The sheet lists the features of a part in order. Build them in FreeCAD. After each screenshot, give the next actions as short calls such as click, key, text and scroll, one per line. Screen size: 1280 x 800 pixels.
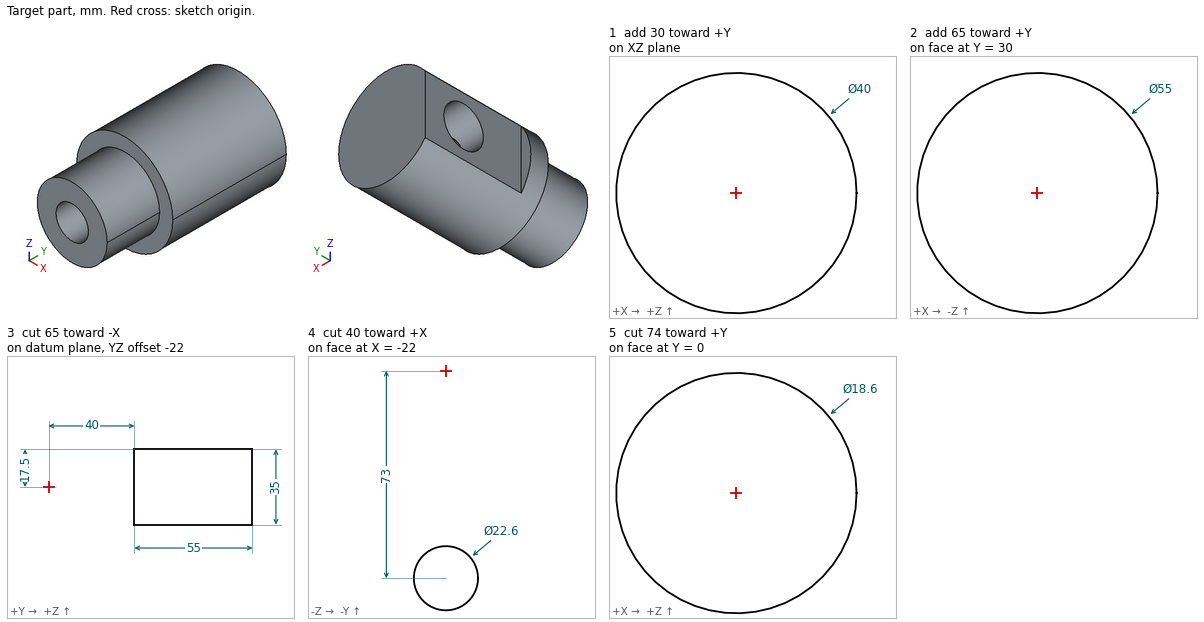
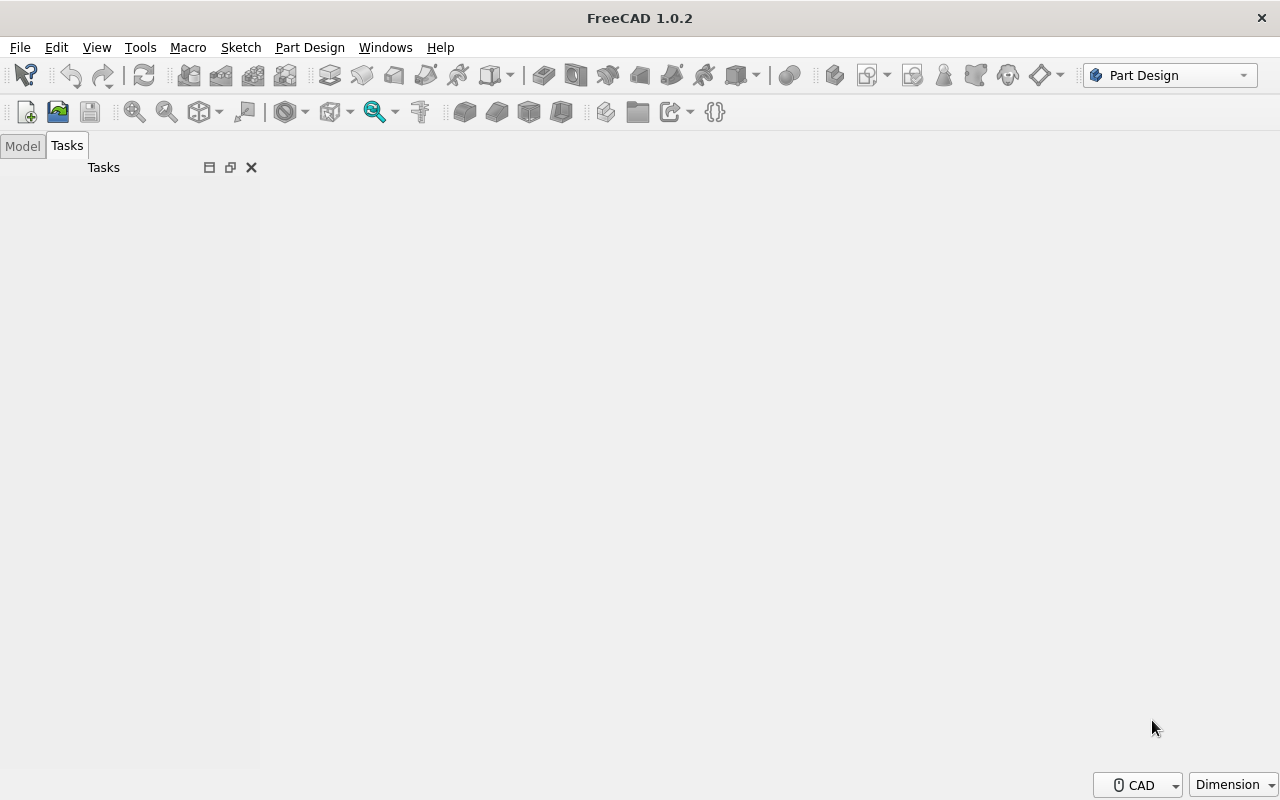
key(ctrl+n)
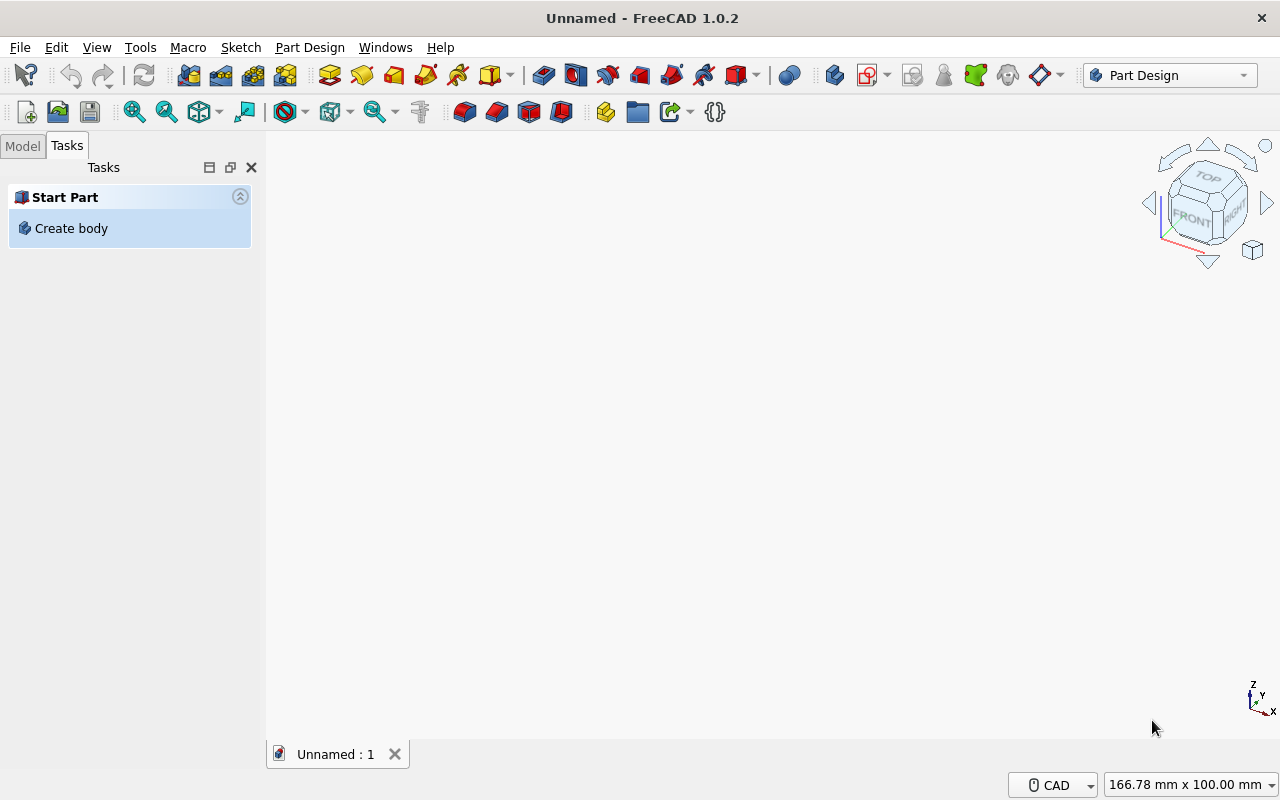
click(868, 76)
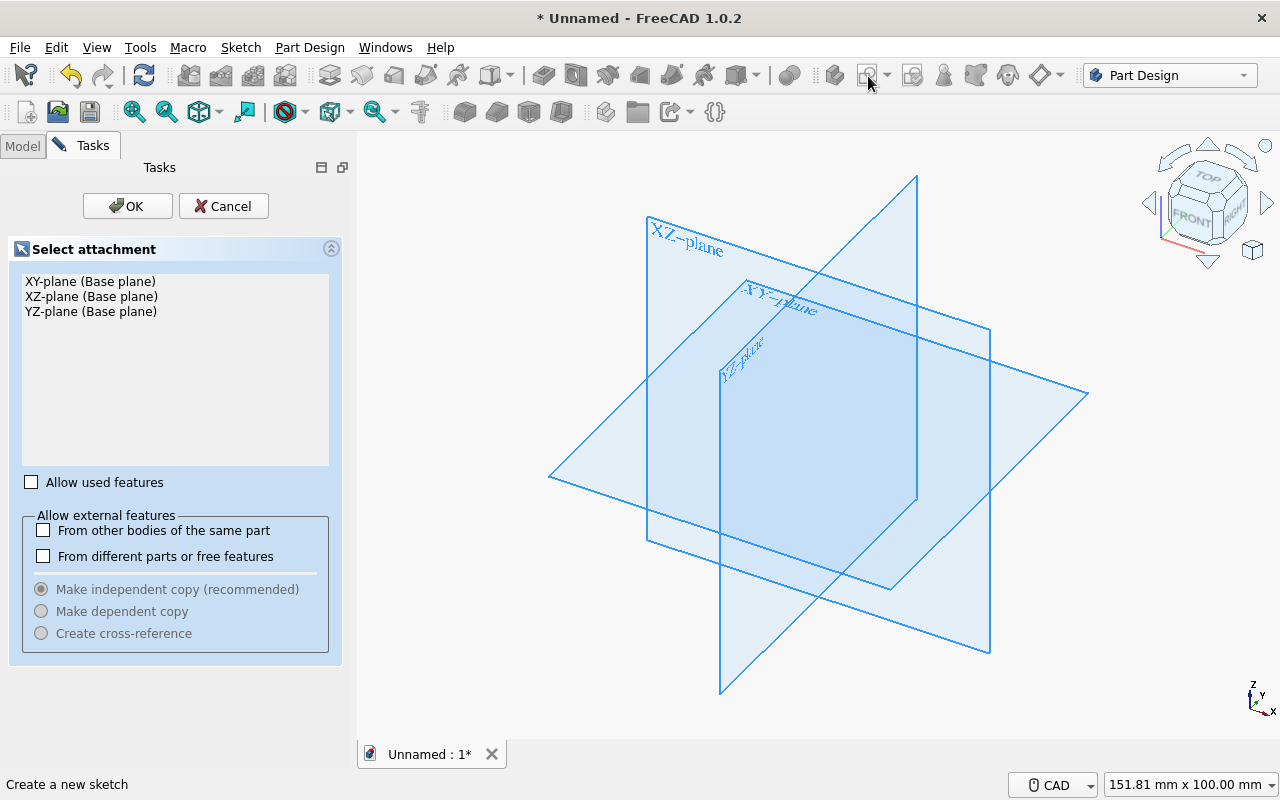
click(82, 296)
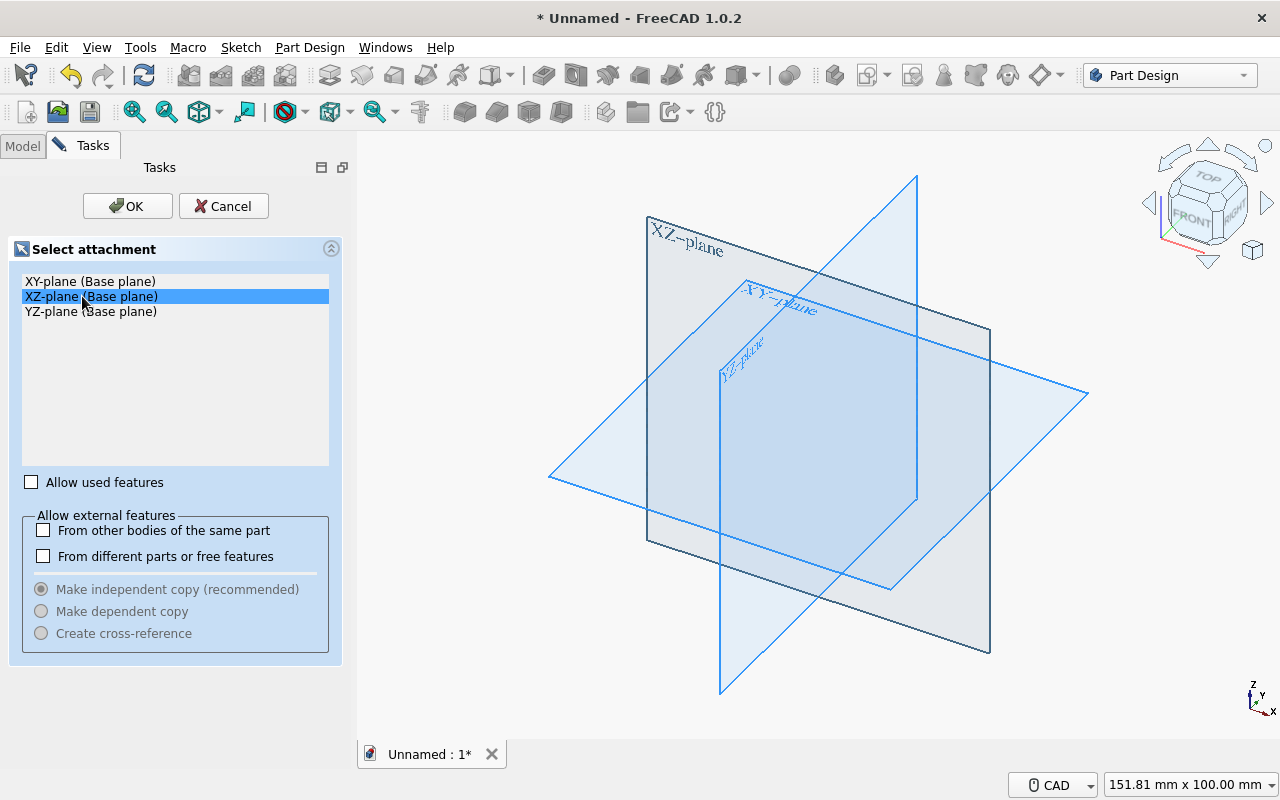
click(128, 206)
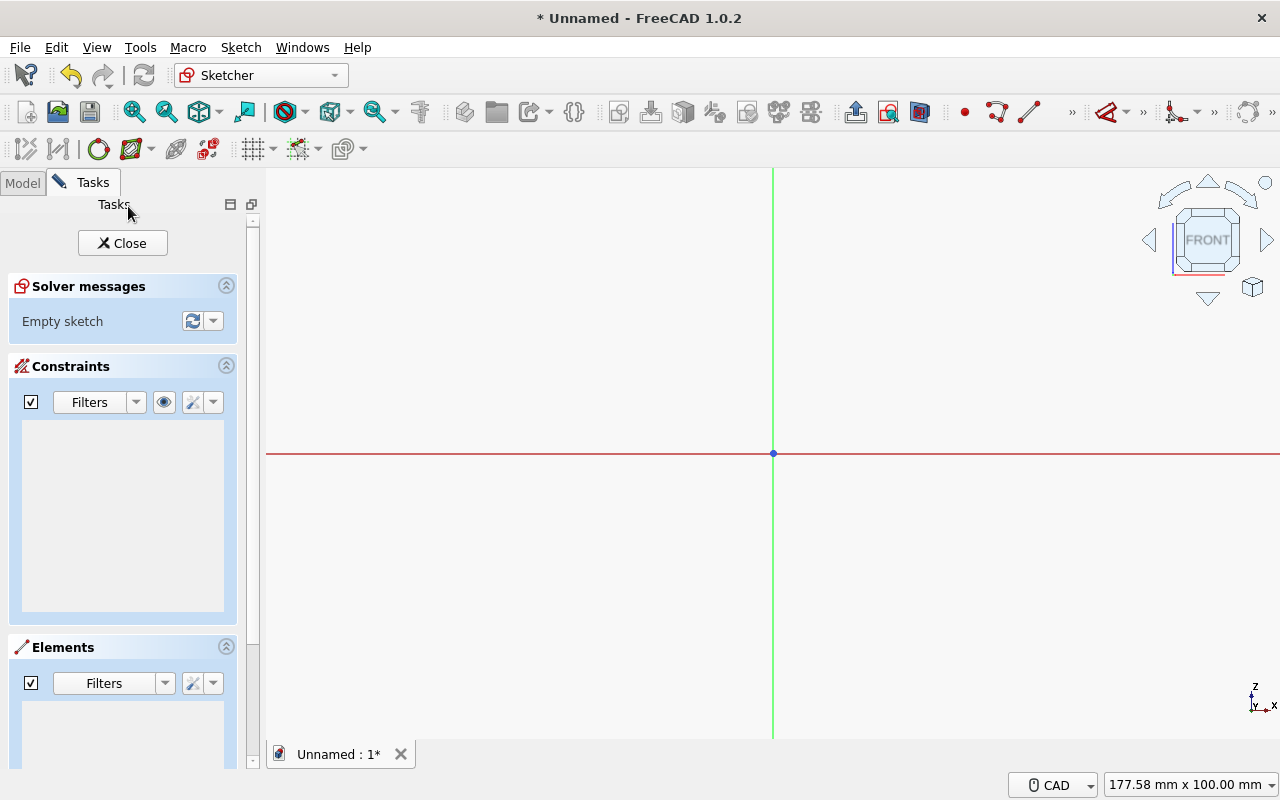
scroll(912, 454, up, 2)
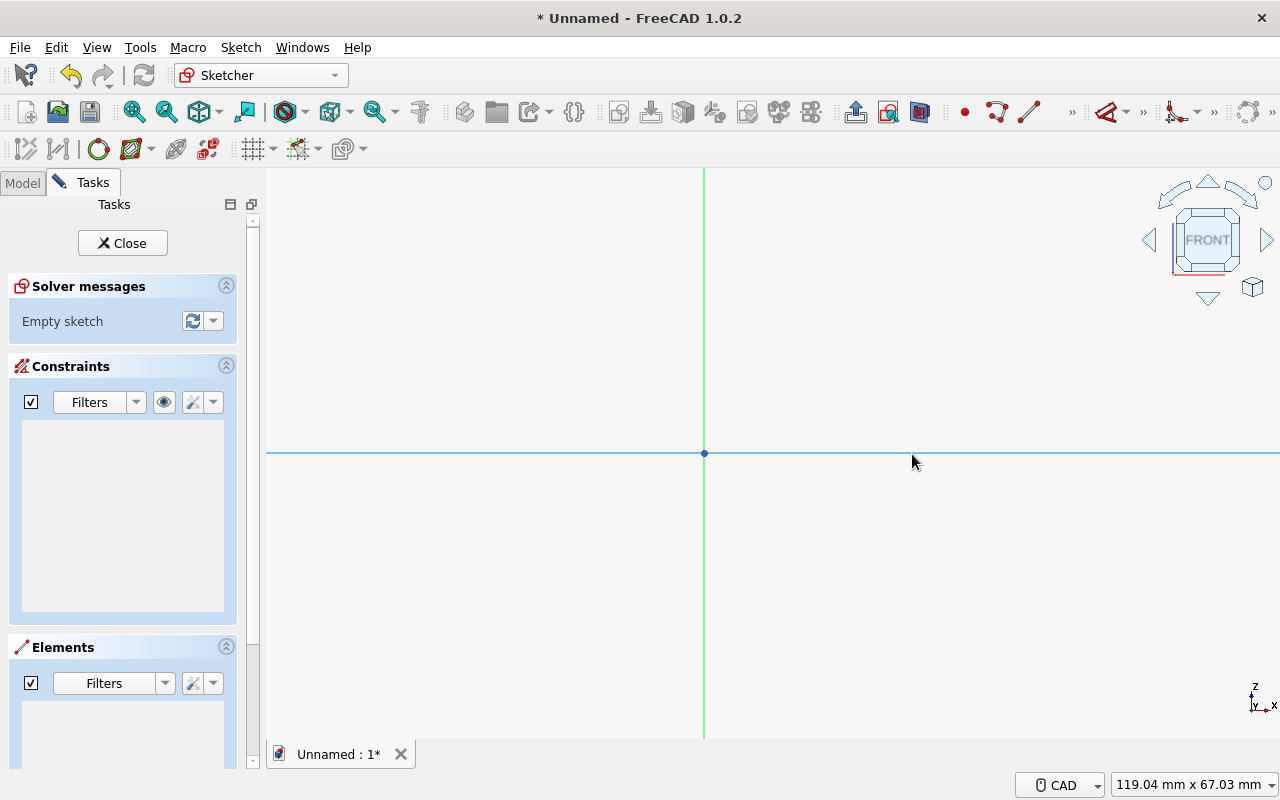
key(g)
key(c)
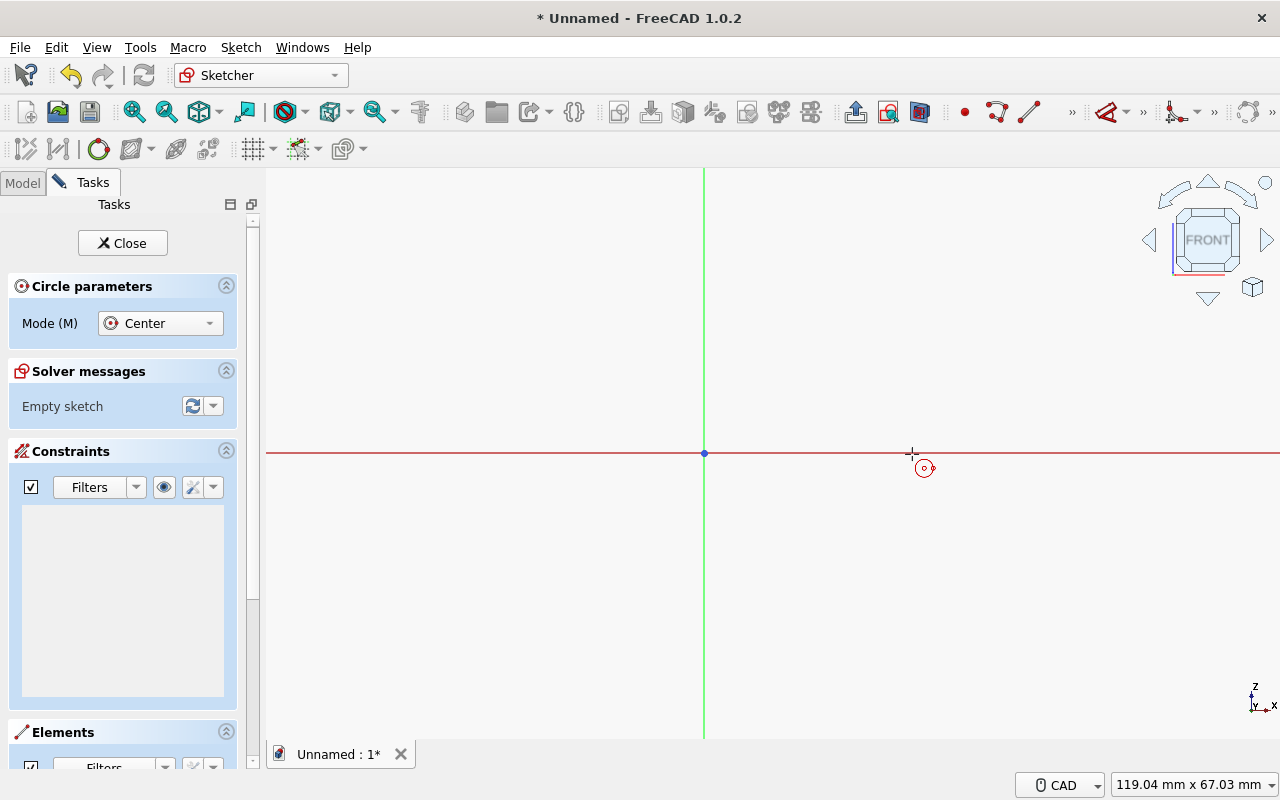
click(704, 453)
move(825, 333)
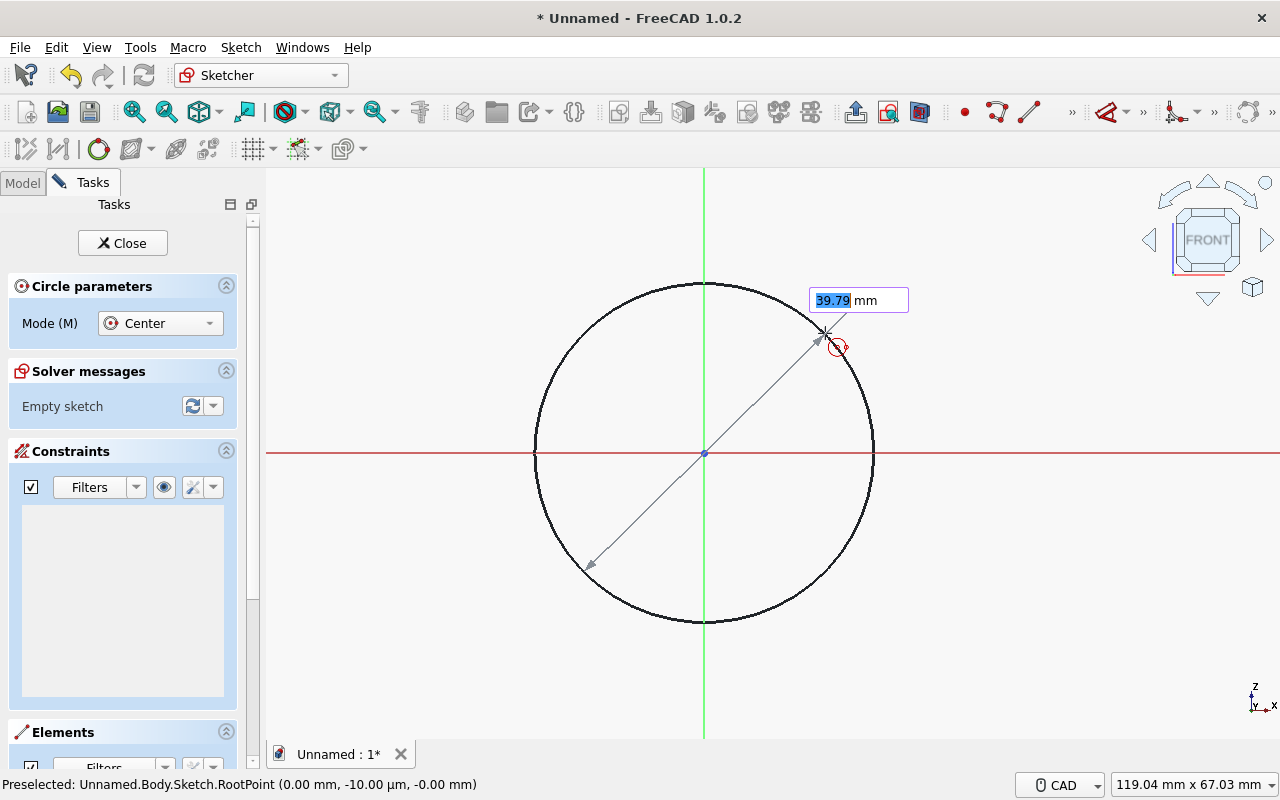
text(40)
key(Return)
key(Escape)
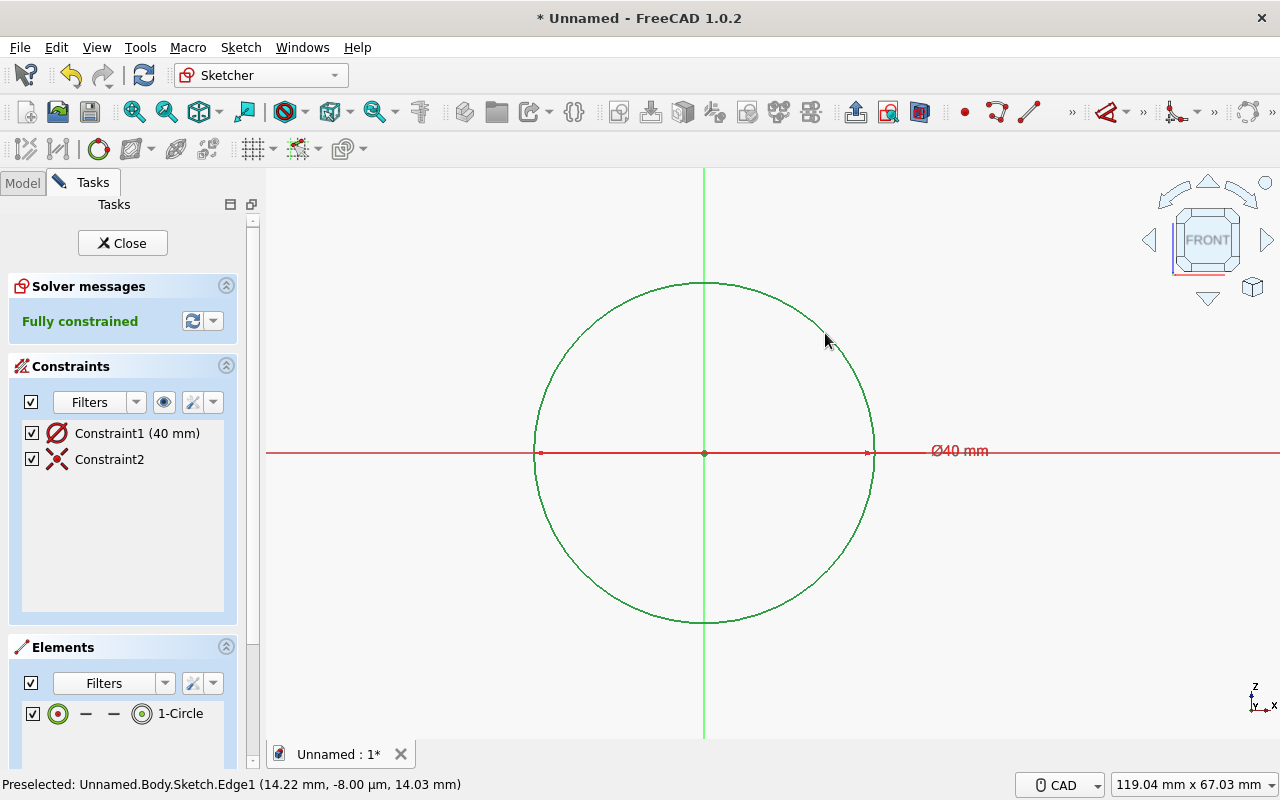
click(123, 243)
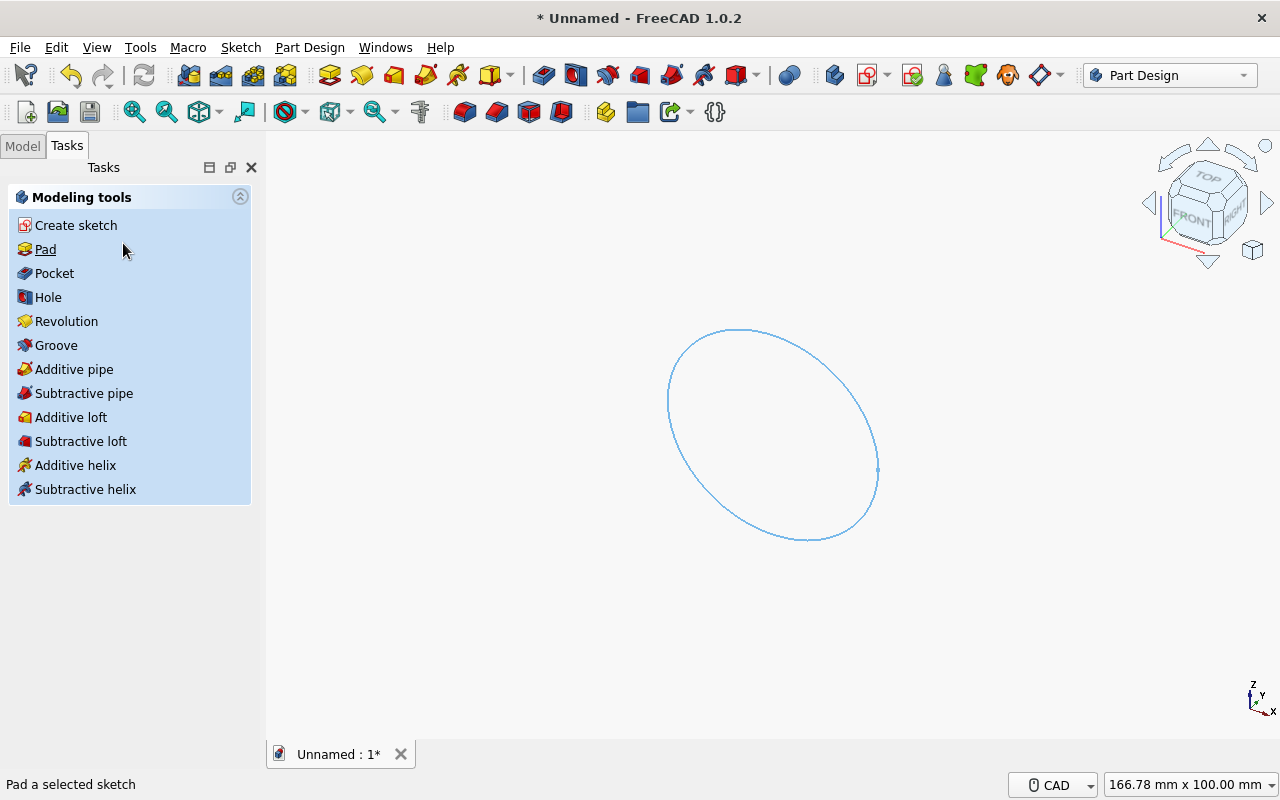
click(330, 76)